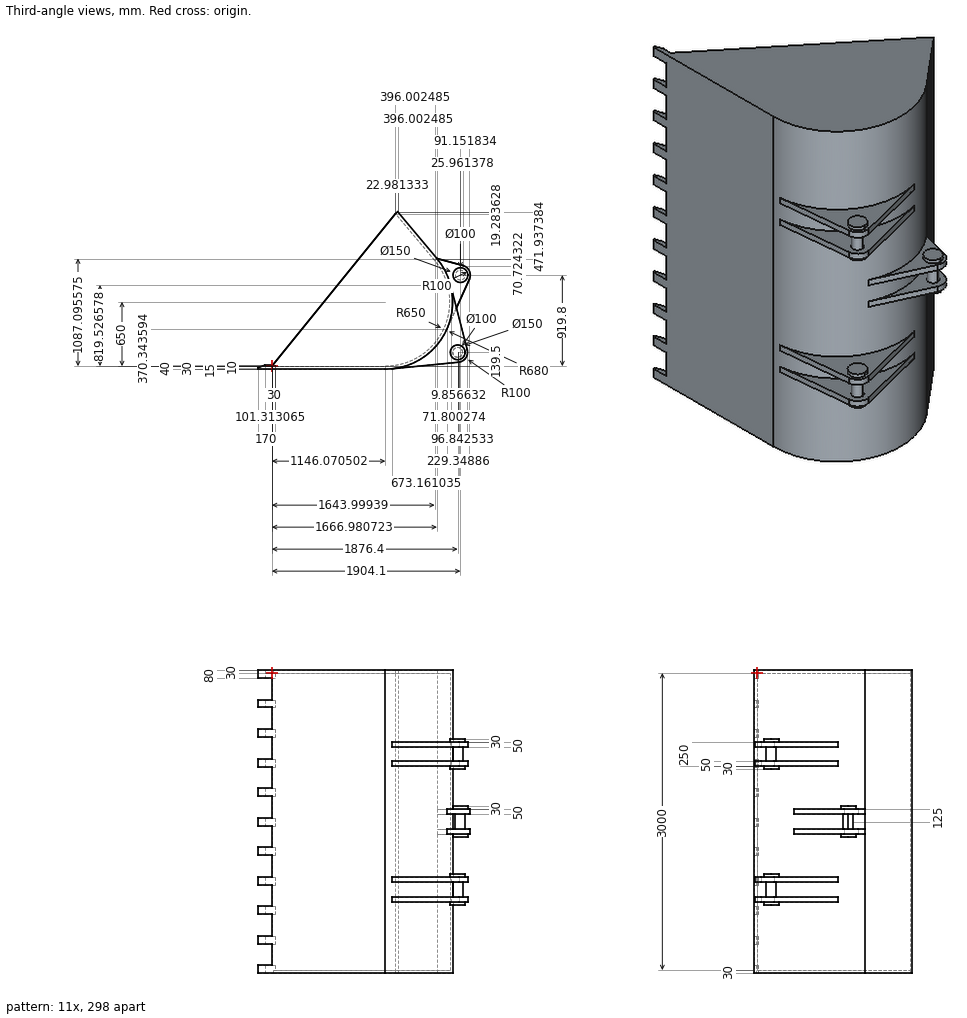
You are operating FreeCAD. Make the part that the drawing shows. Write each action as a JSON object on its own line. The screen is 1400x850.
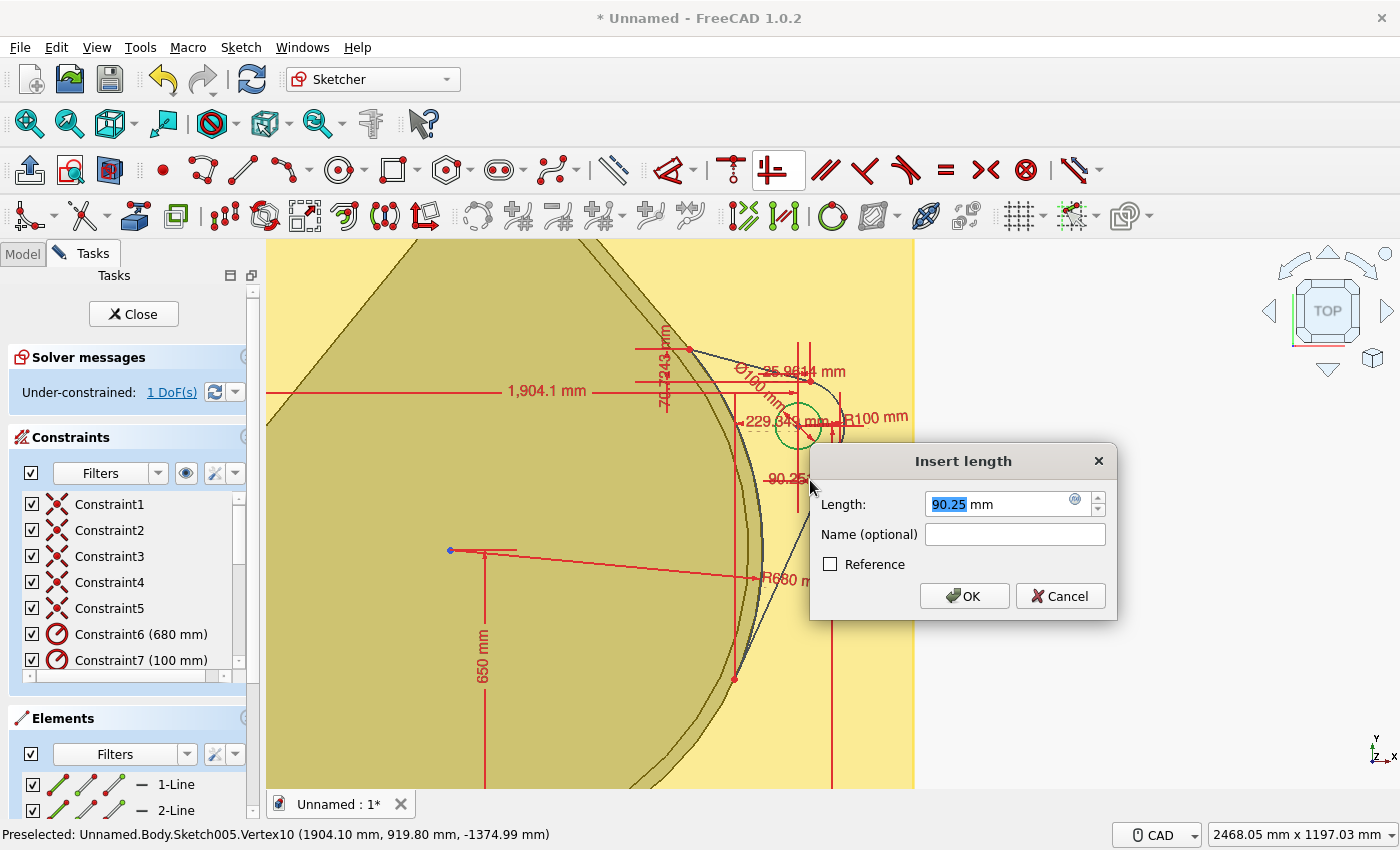
{"action": "type", "text": "91.151834"}
{"action": "key", "text": "Return"}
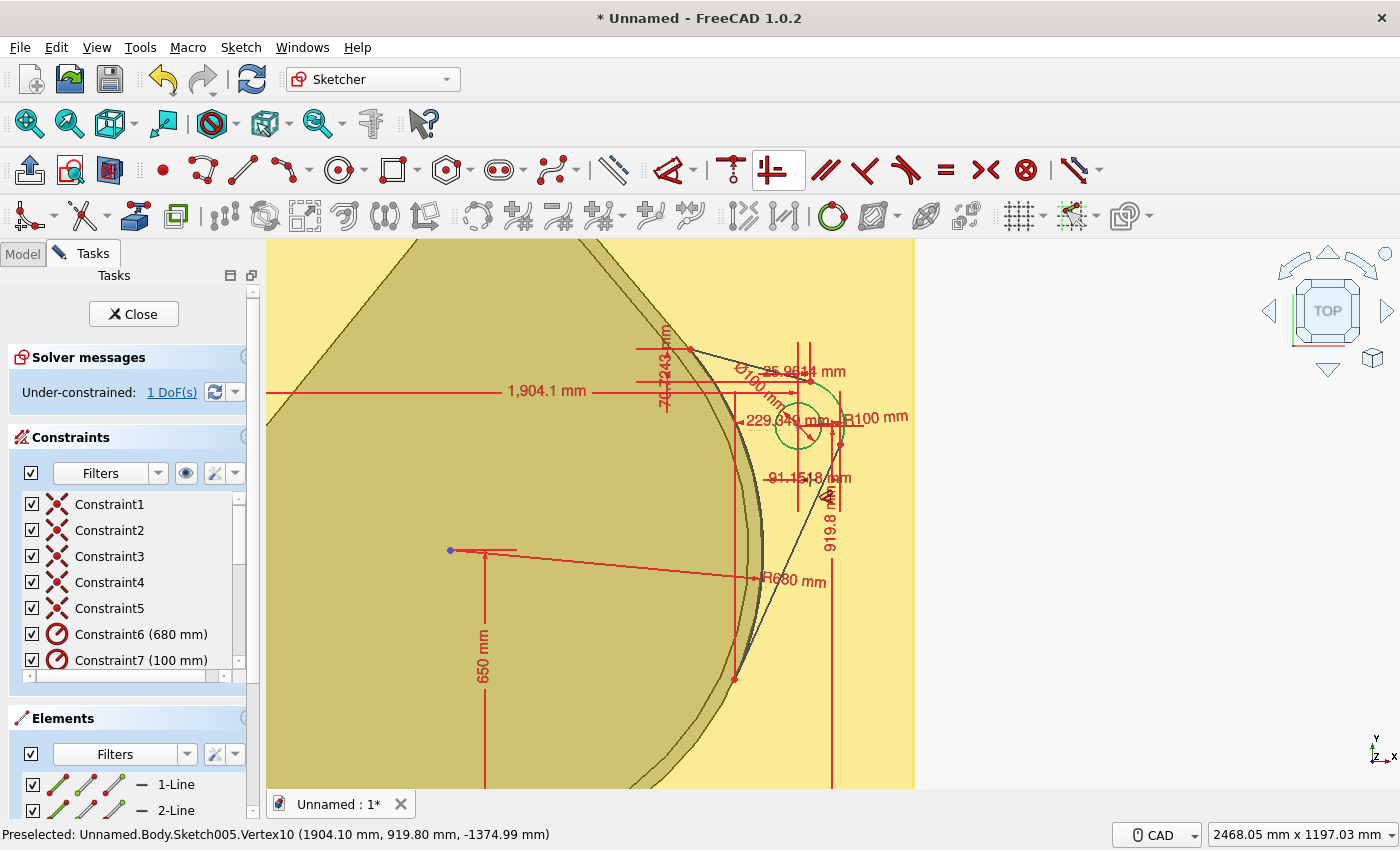
{"action": "left_click", "coordinate": [735, 680]}
{"action": "left_click", "coordinate": [769, 720]}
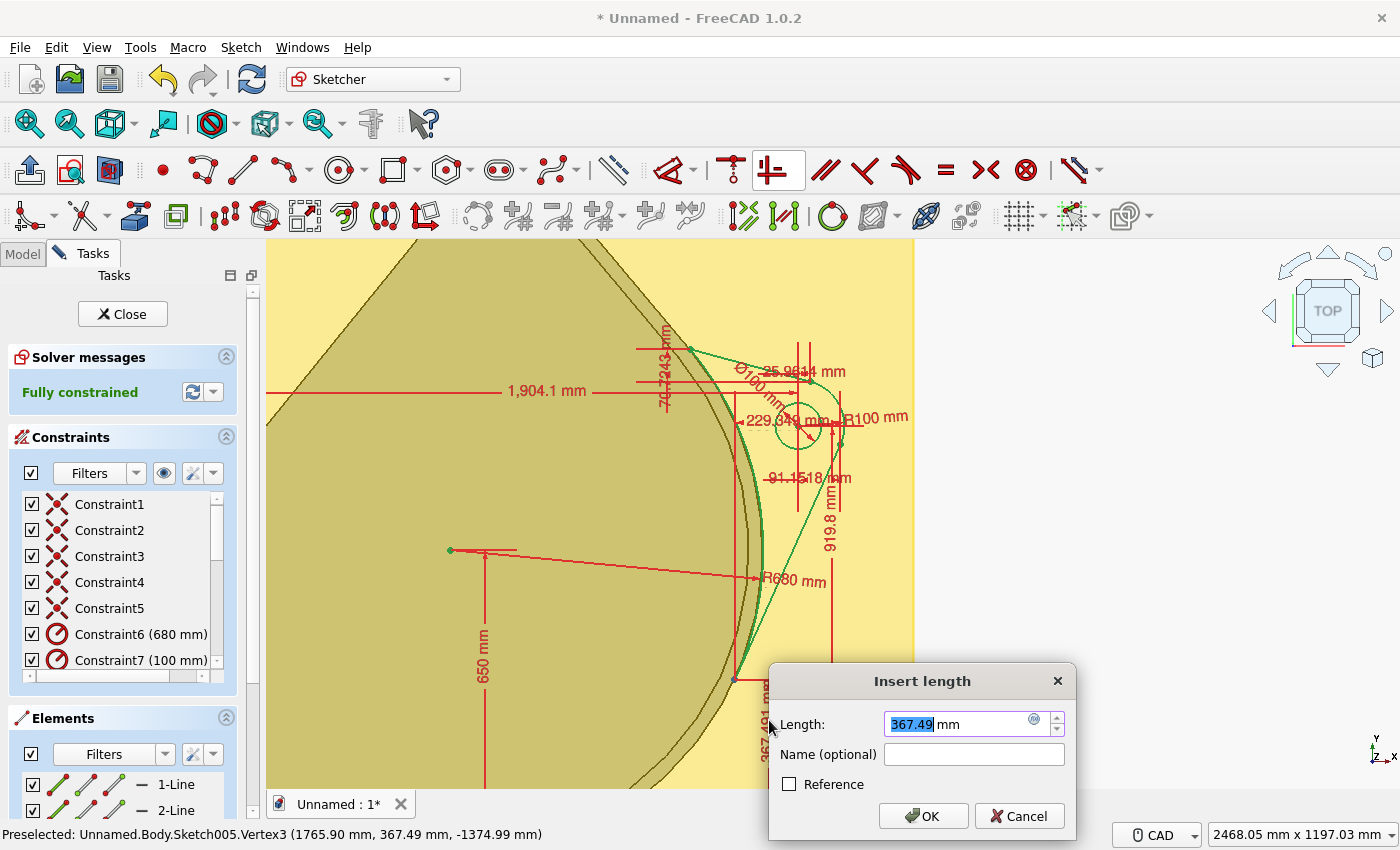
{"action": "type", "text": "370.343594"}
{"action": "key", "text": "Return"}
{"action": "key", "text": "Escape"}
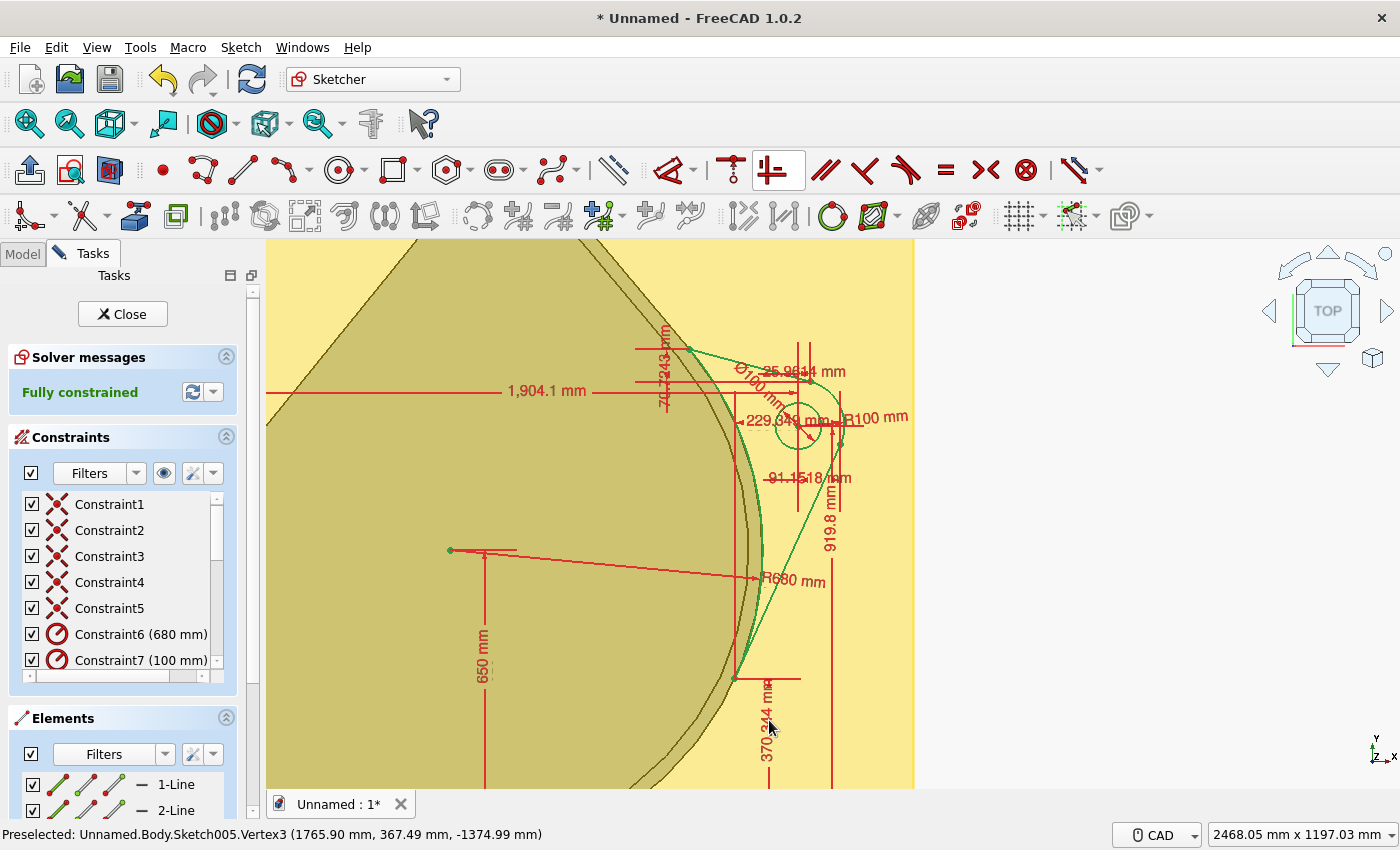
{"action": "left_click", "coordinate": [123, 314]}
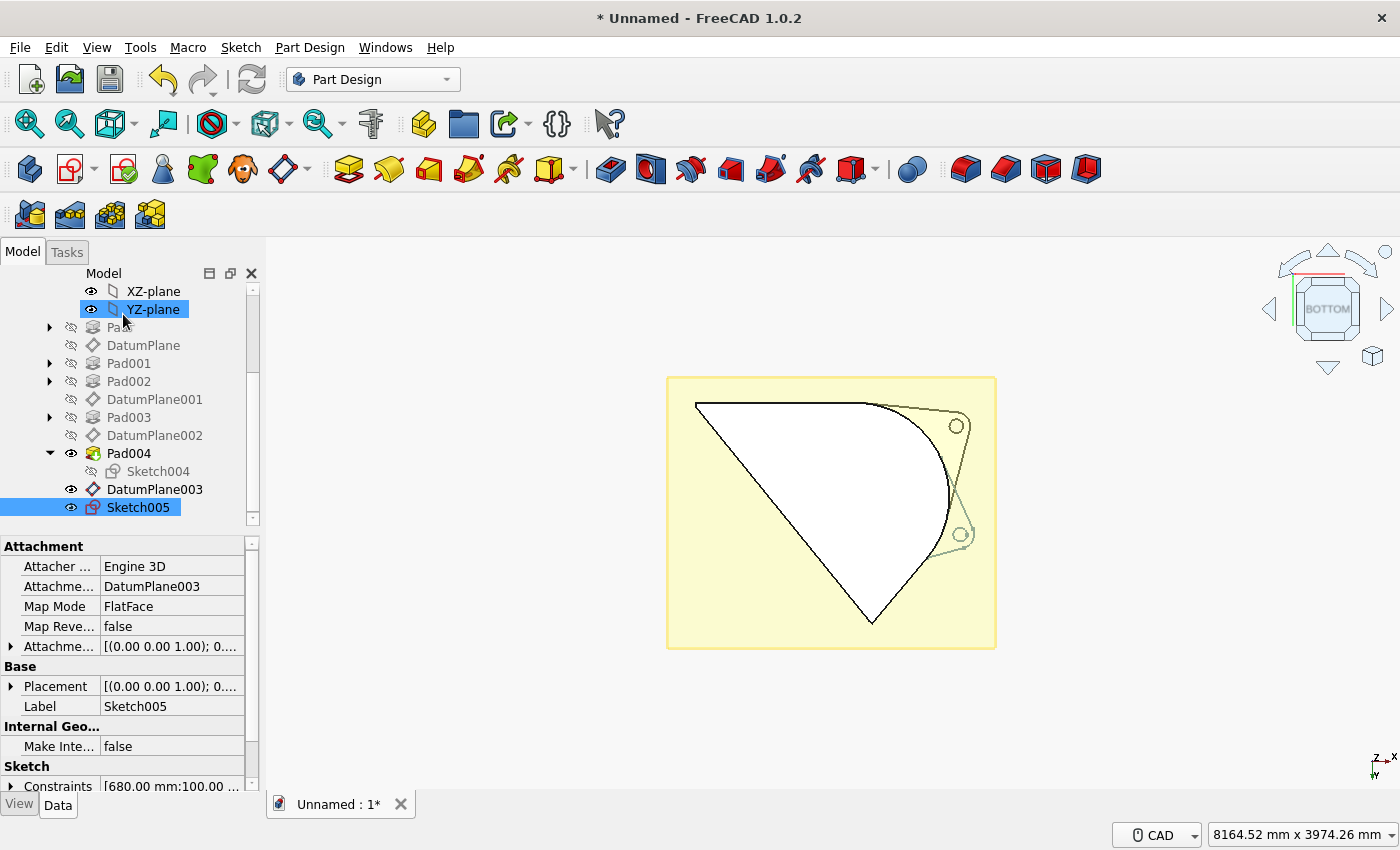
{"action": "left_click", "coordinate": [350, 170]}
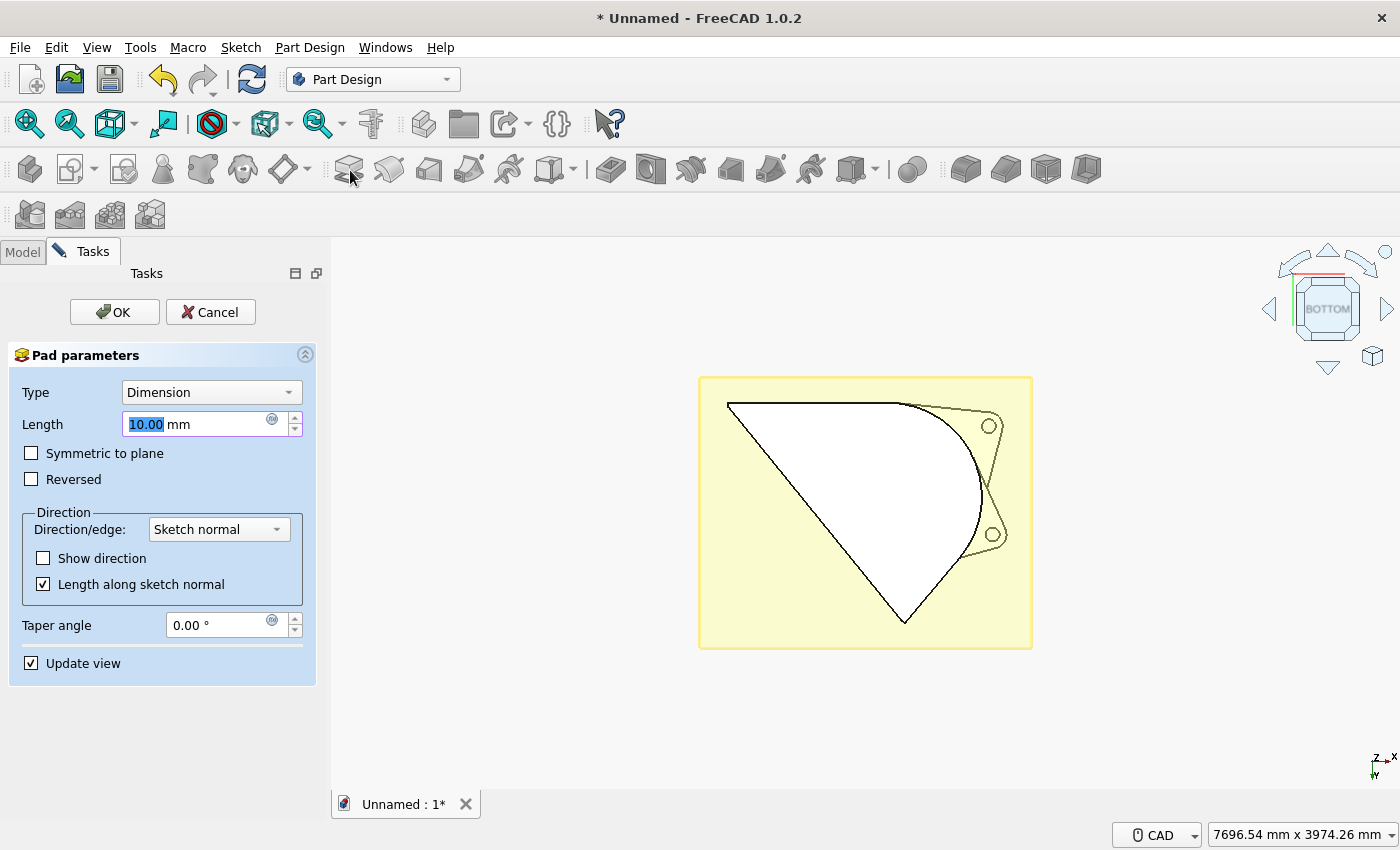
{"action": "type", "text": "50"}
{"action": "key", "text": "Tab"}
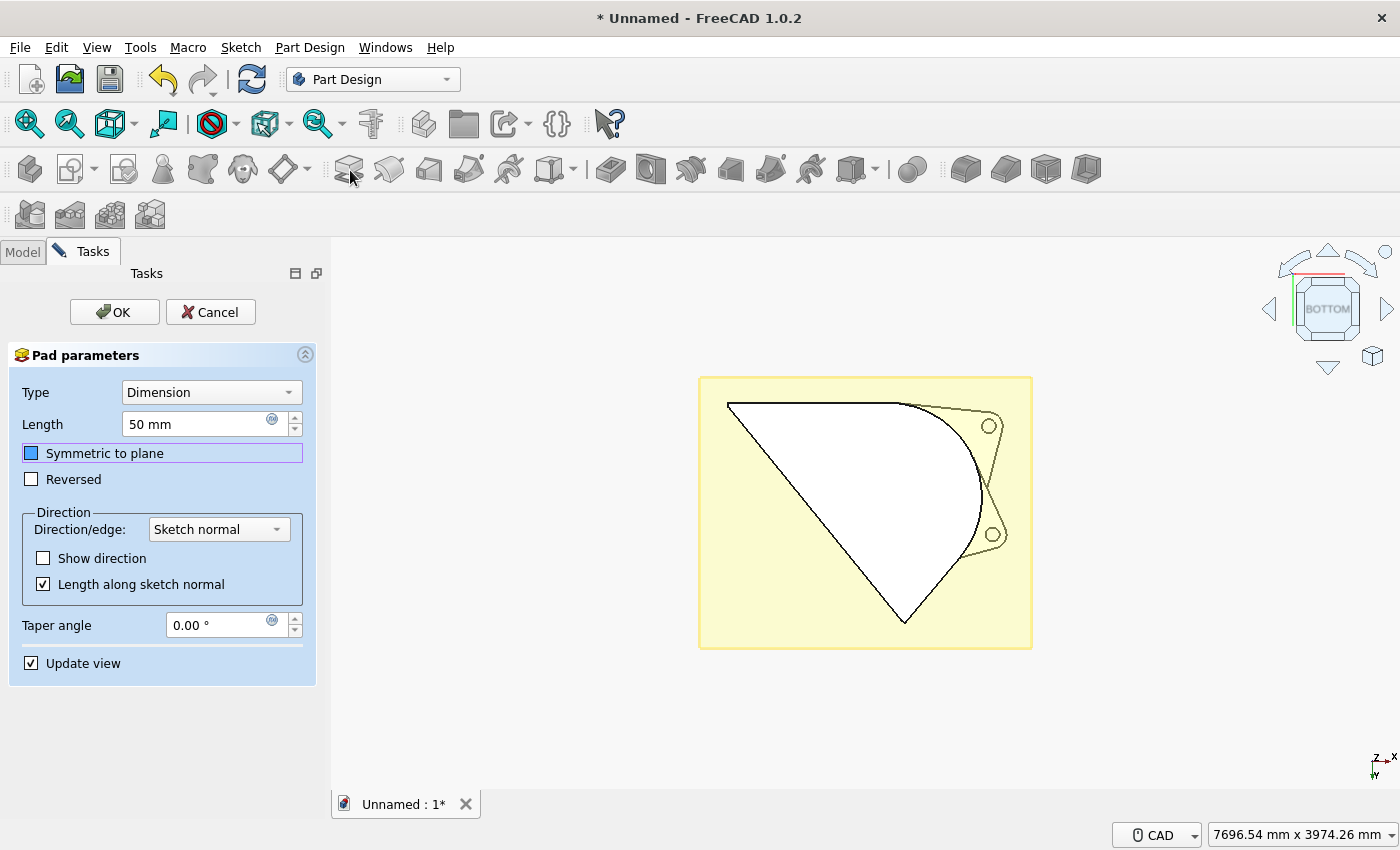
{"action": "left_click", "coordinate": [30, 479]}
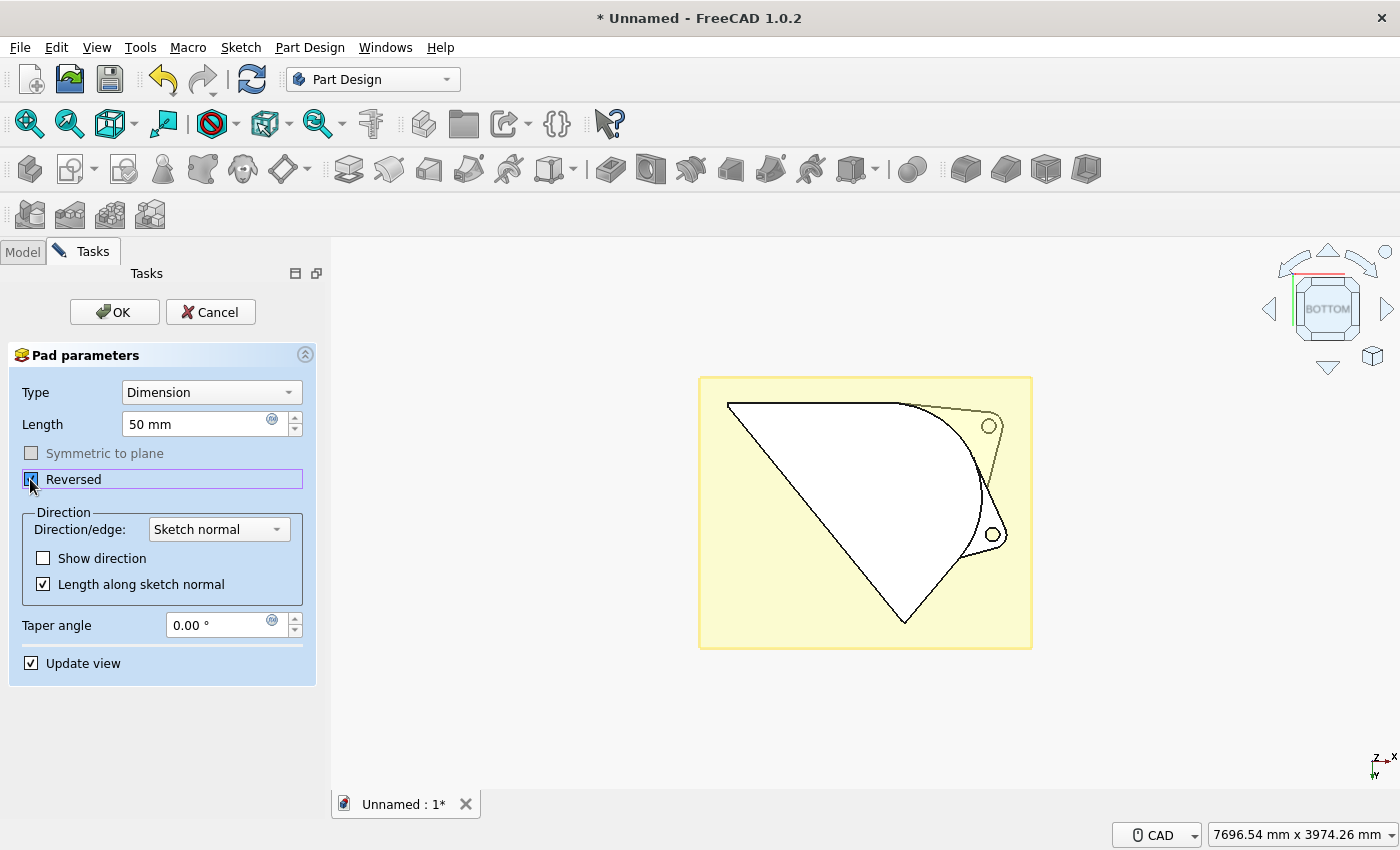
{"action": "left_click", "coordinate": [115, 312]}